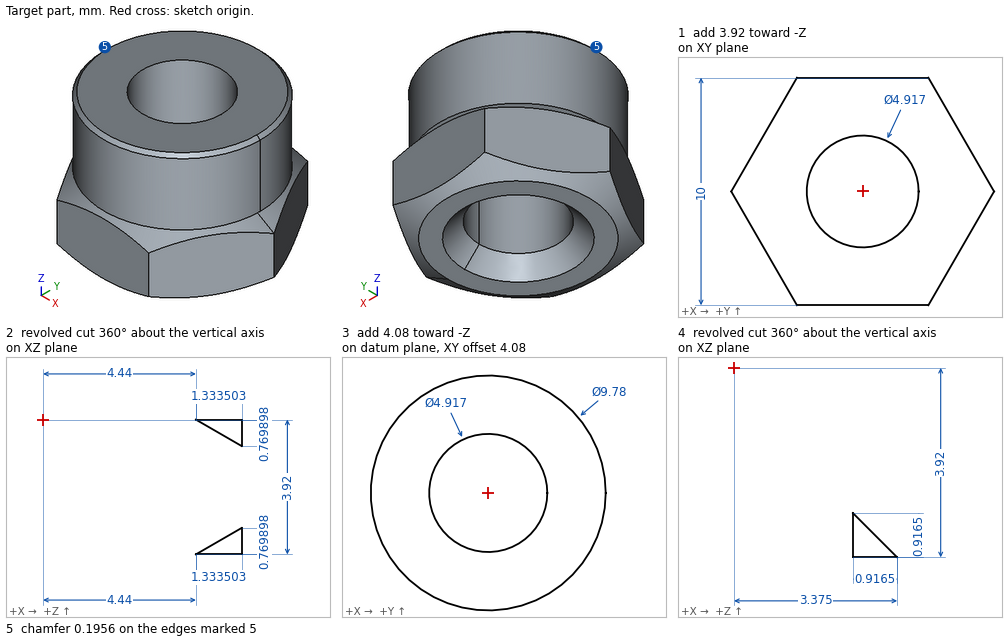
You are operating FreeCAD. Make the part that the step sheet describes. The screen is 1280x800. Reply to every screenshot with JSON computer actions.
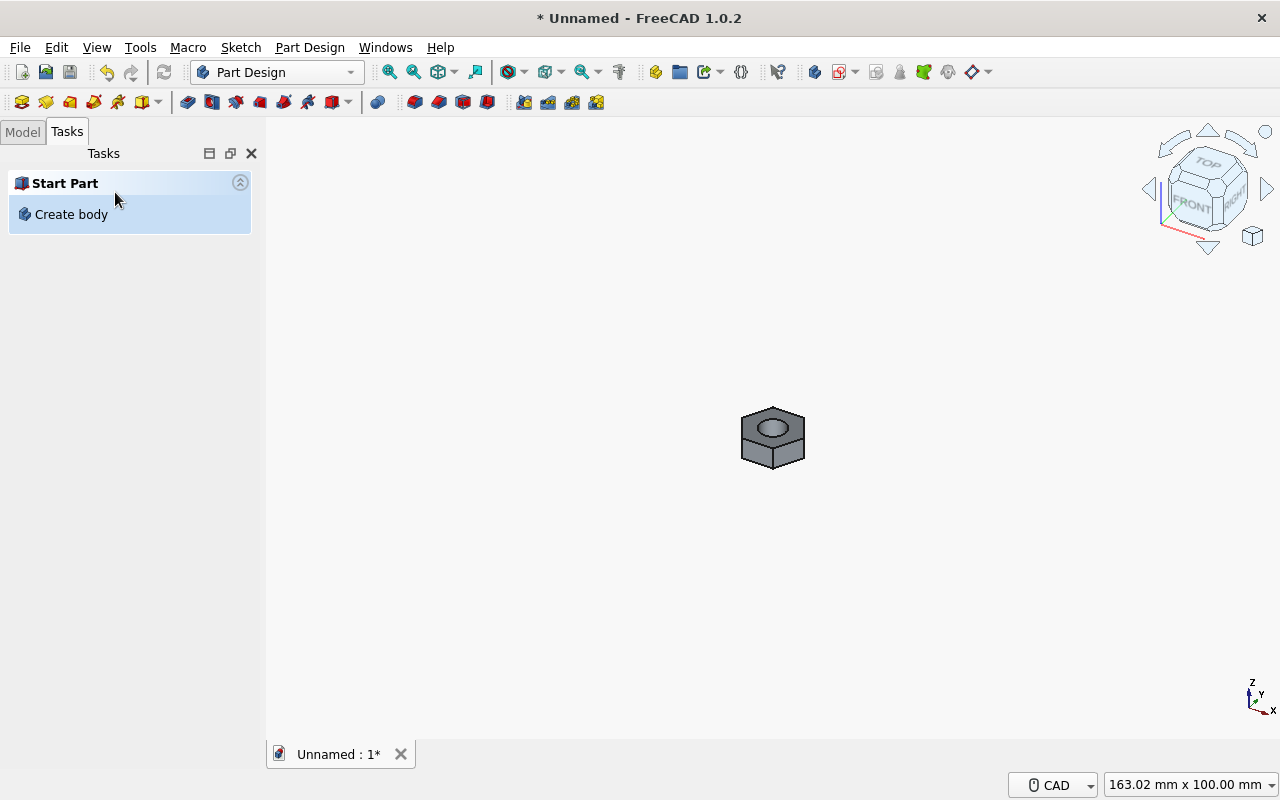
{"action": "key", "text": "v f"}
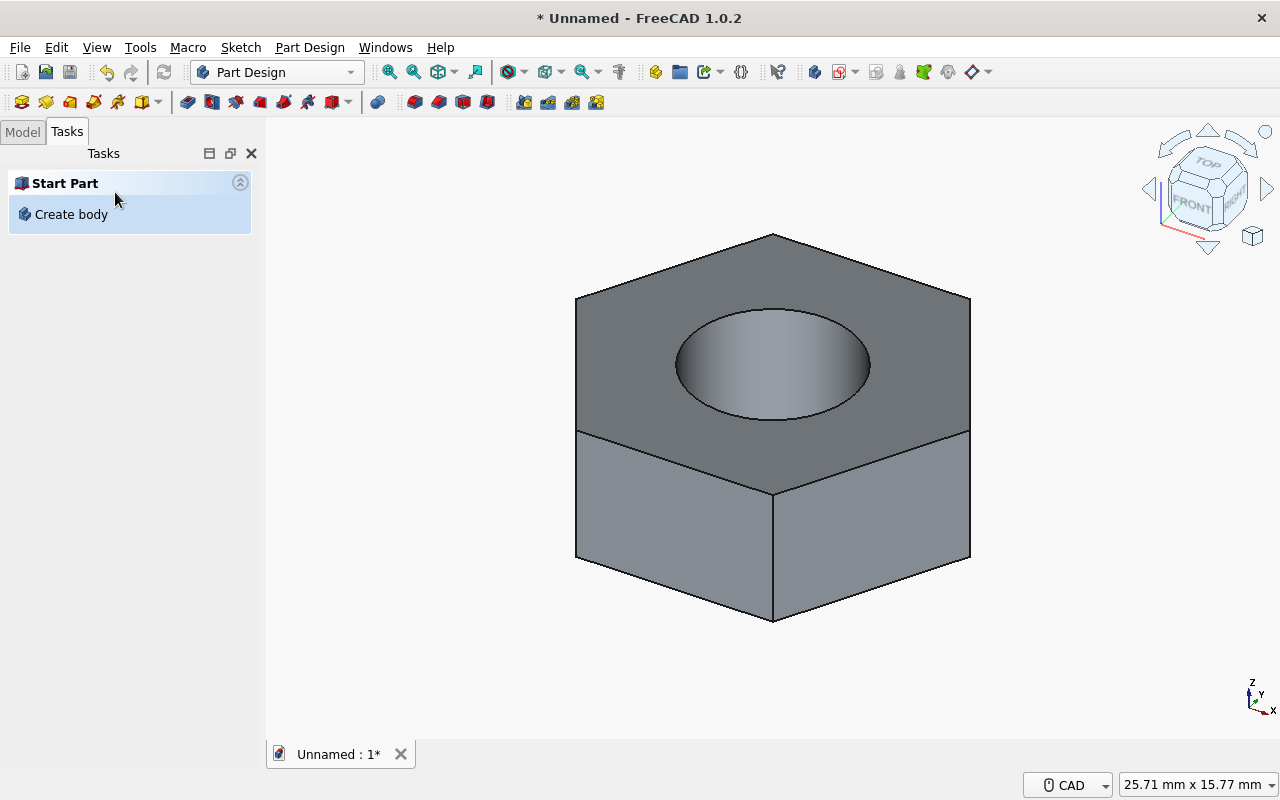
{"action": "left_click", "coordinate": [840, 72]}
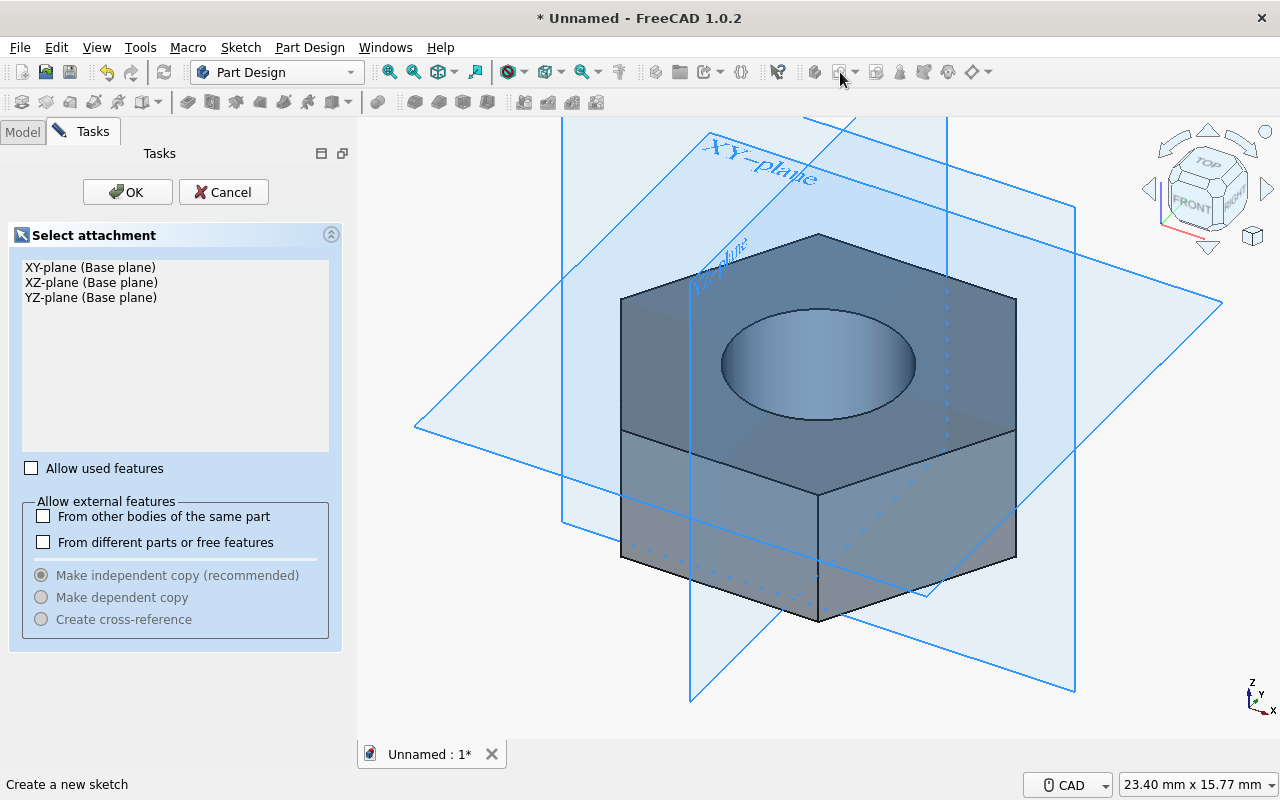
{"action": "left_click", "coordinate": [82, 282]}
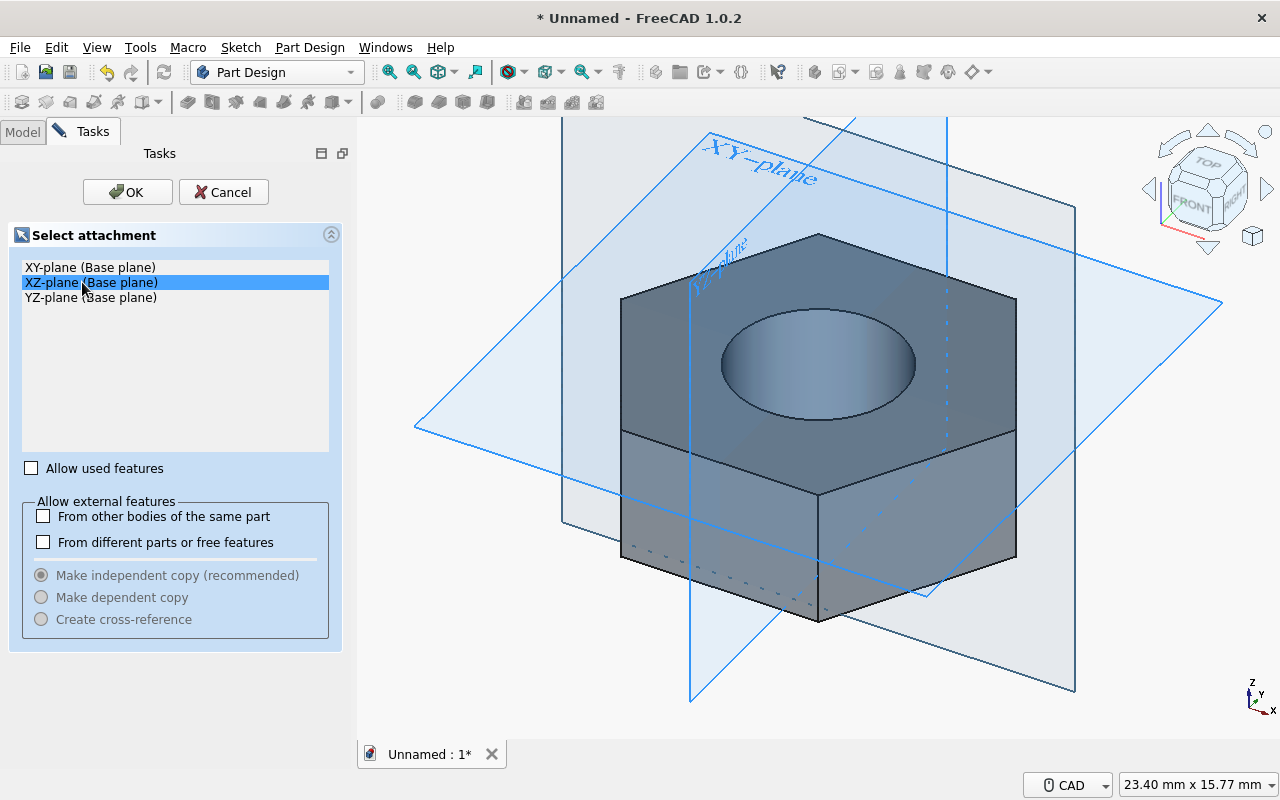
{"action": "left_click", "coordinate": [128, 192]}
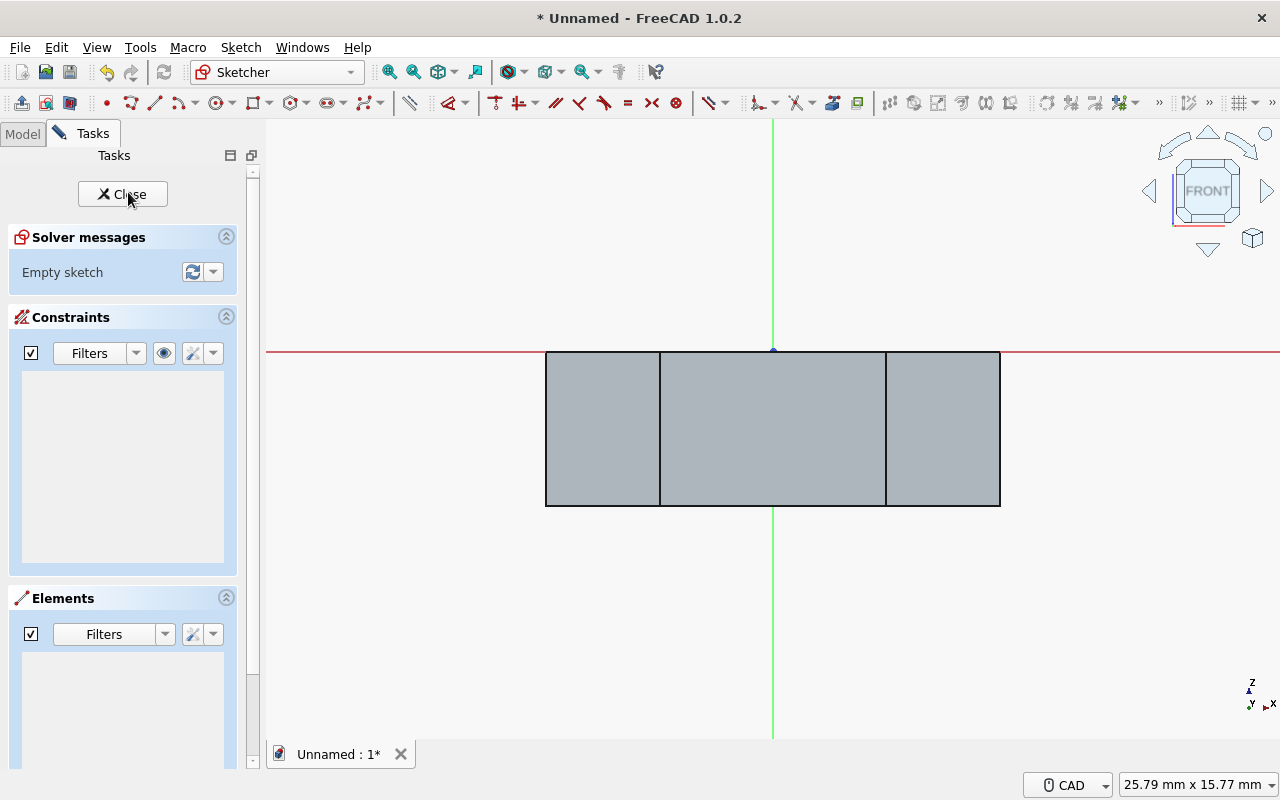
{"action": "key", "text": "q s"}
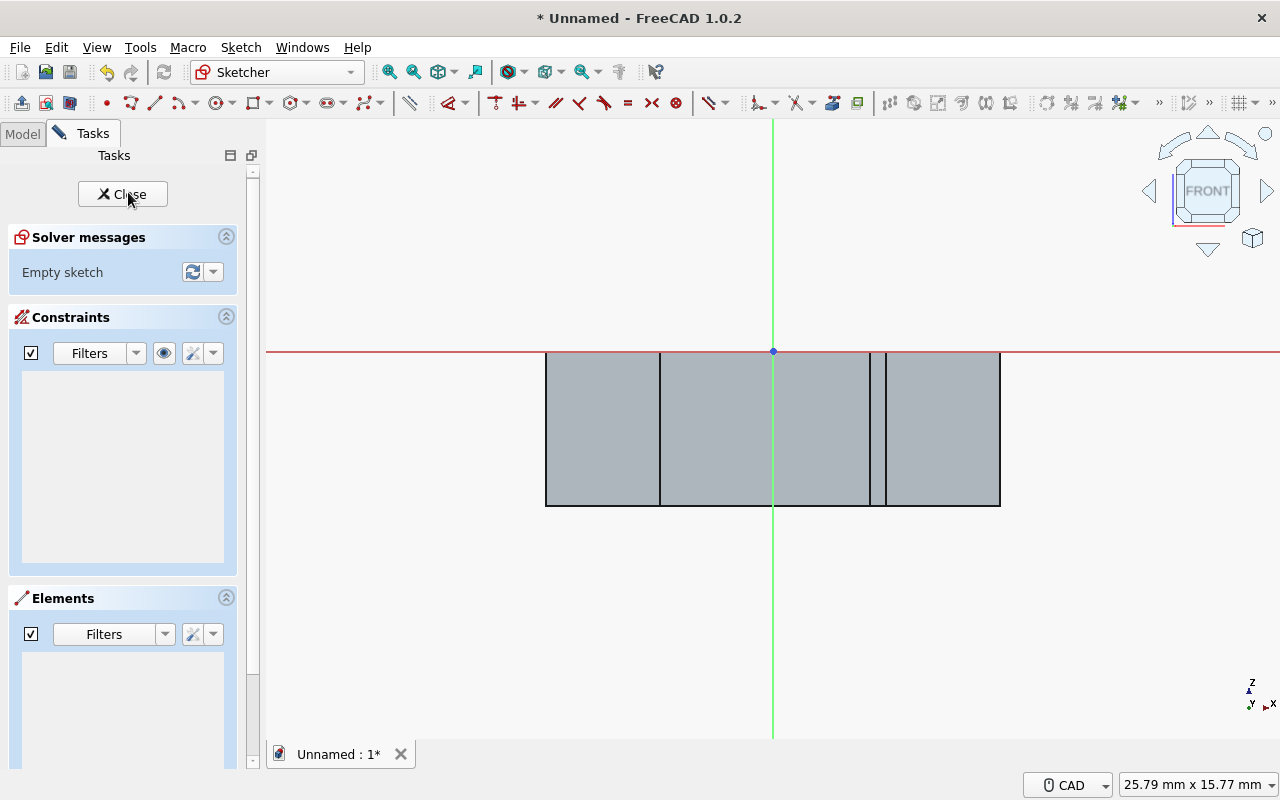
{"action": "scroll", "coordinate": [992, 429], "scroll_direction": "up", "scroll_amount": 5}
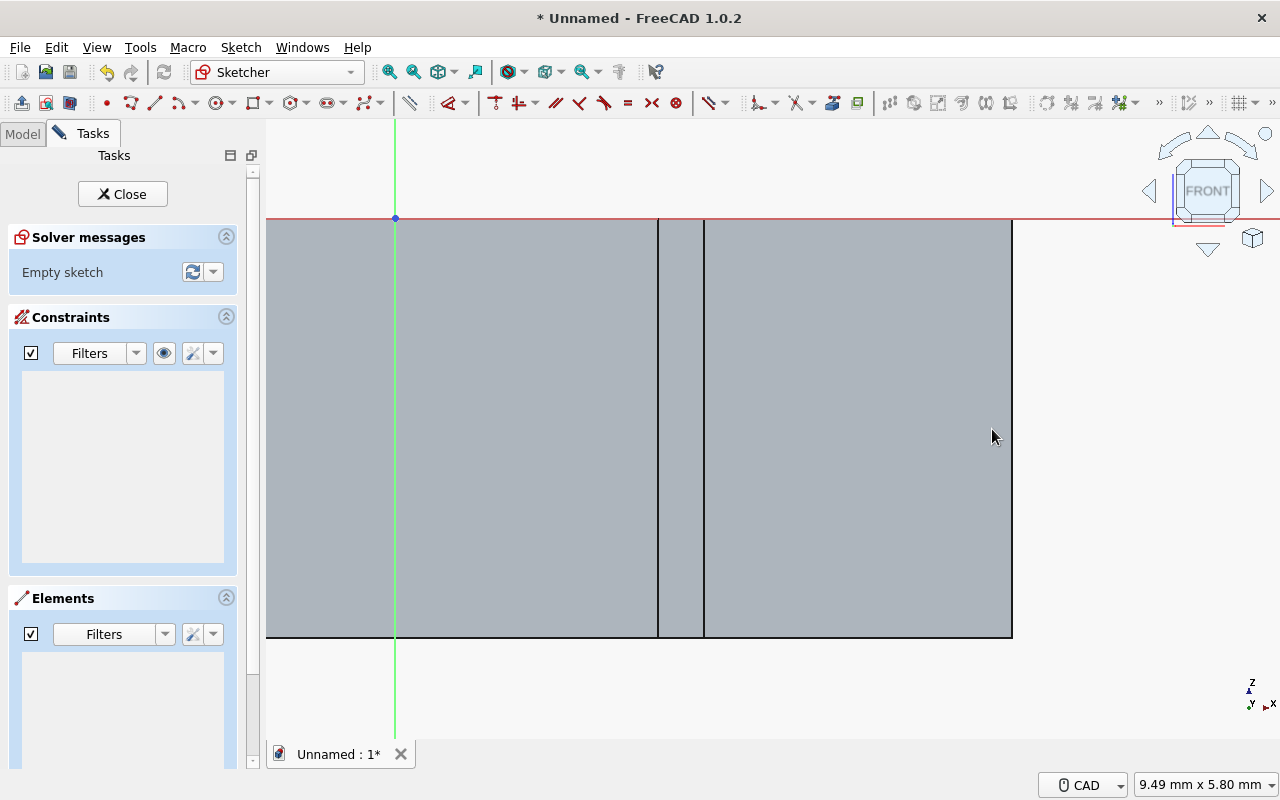
{"action": "key", "text": "g m"}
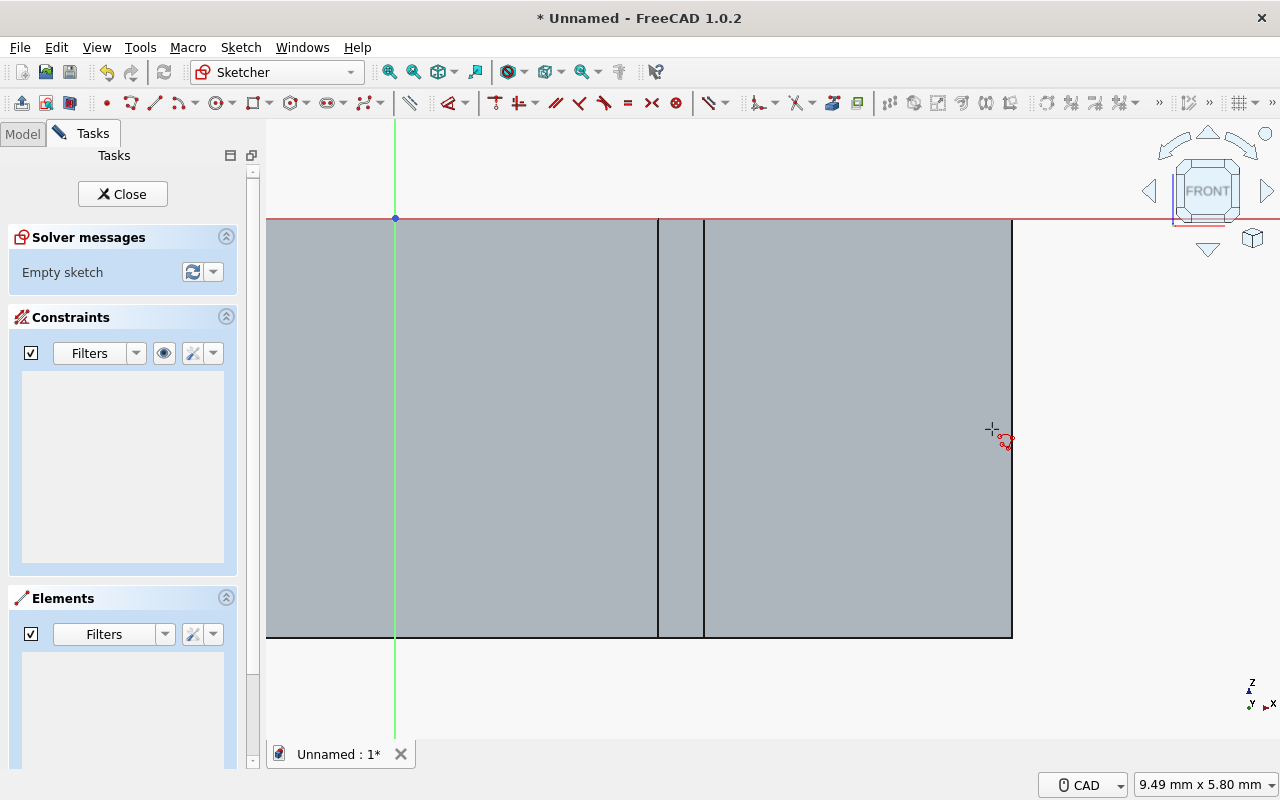
{"action": "left_click", "coordinate": [870, 638]}
{"action": "left_click", "coordinate": [1012, 555]}
{"action": "left_click", "coordinate": [1012, 638]}
{"action": "left_click", "coordinate": [870, 639]}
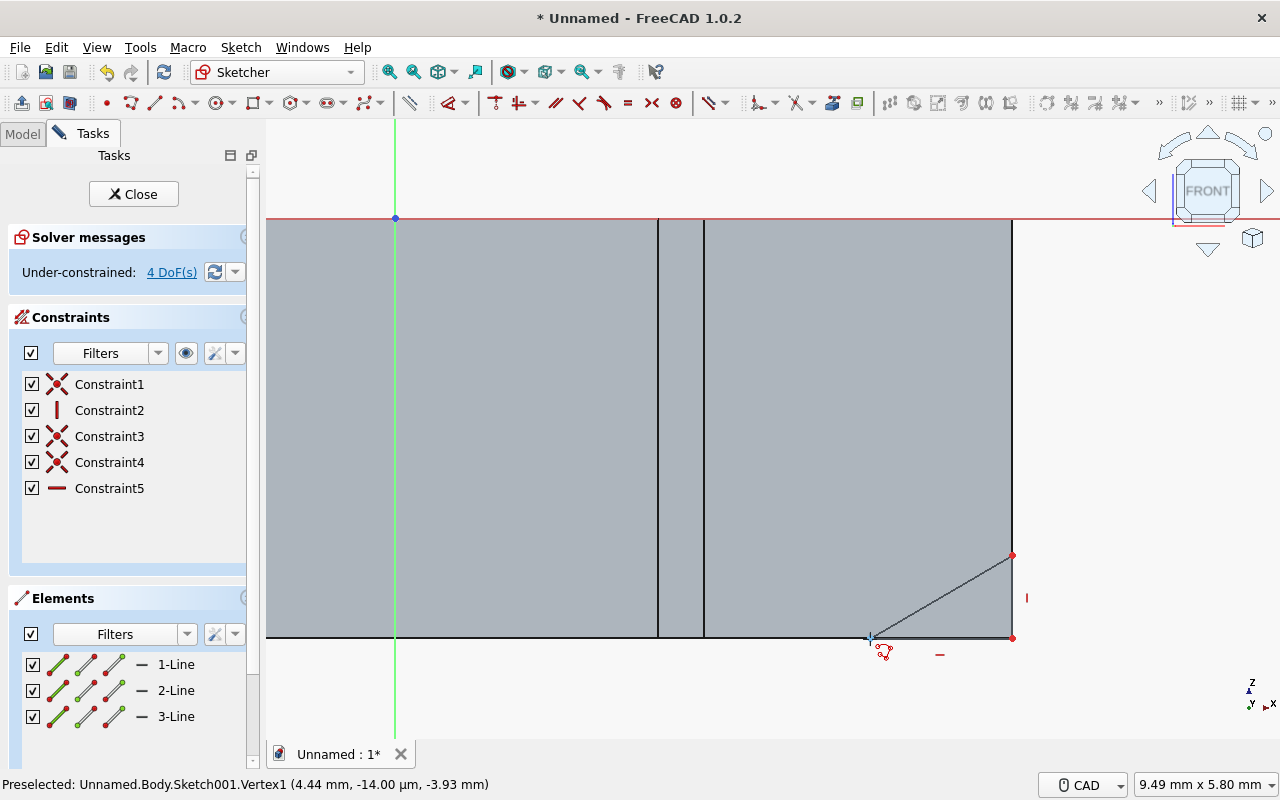
{"action": "left_click", "coordinate": [870, 219]}
{"action": "left_click", "coordinate": [1012, 228]}
{"action": "left_click", "coordinate": [1012, 301]}
{"action": "left_click", "coordinate": [870, 219]}
{"action": "key", "text": "Escape"}
{"action": "key", "text": "Escape"}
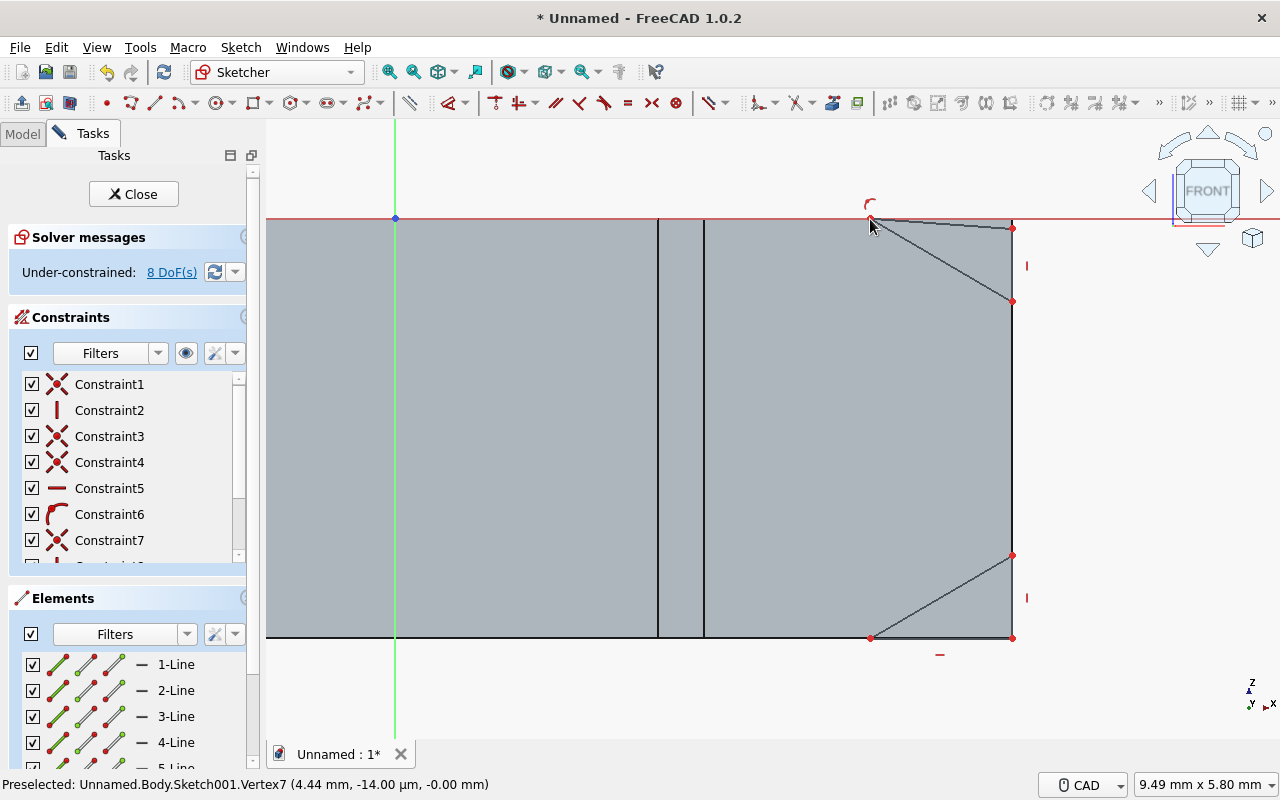
{"action": "left_click", "coordinate": [913, 222]}